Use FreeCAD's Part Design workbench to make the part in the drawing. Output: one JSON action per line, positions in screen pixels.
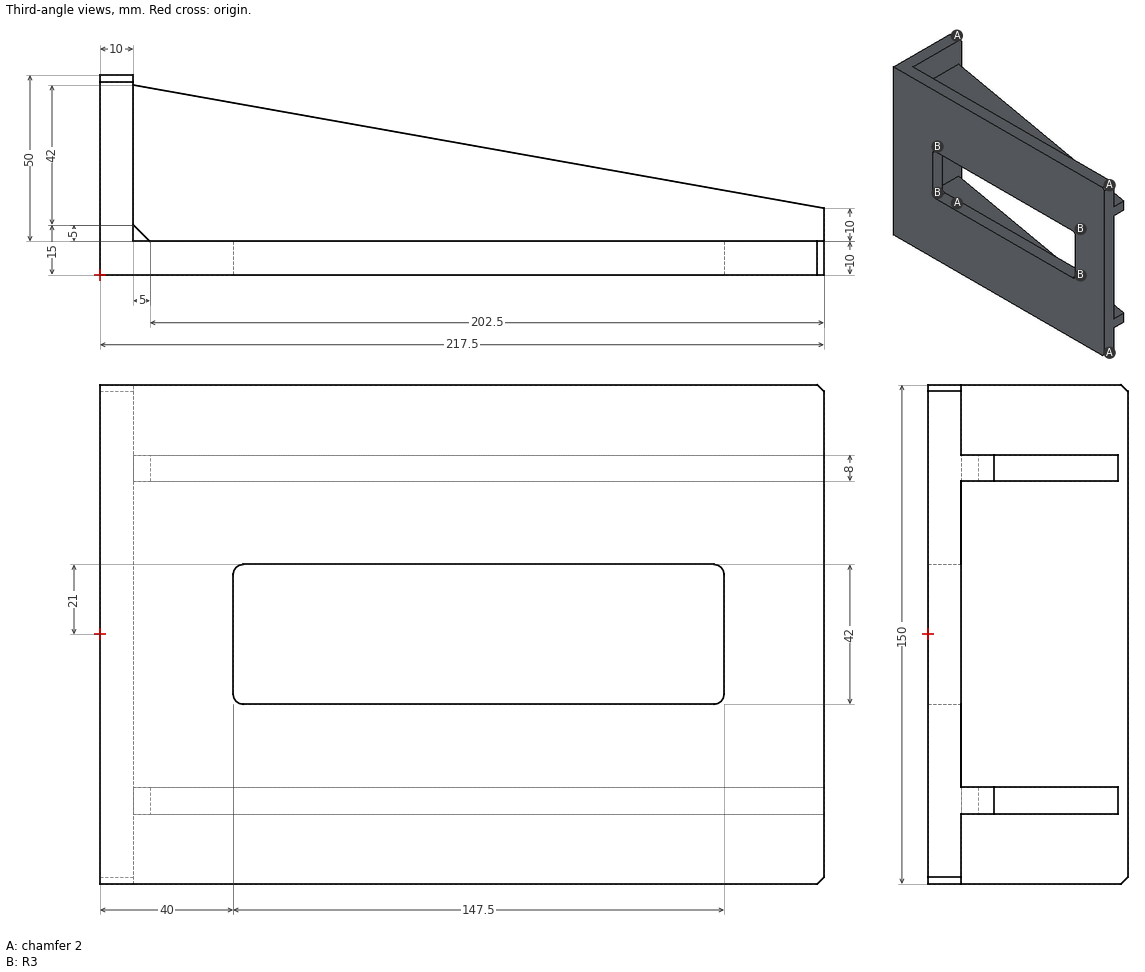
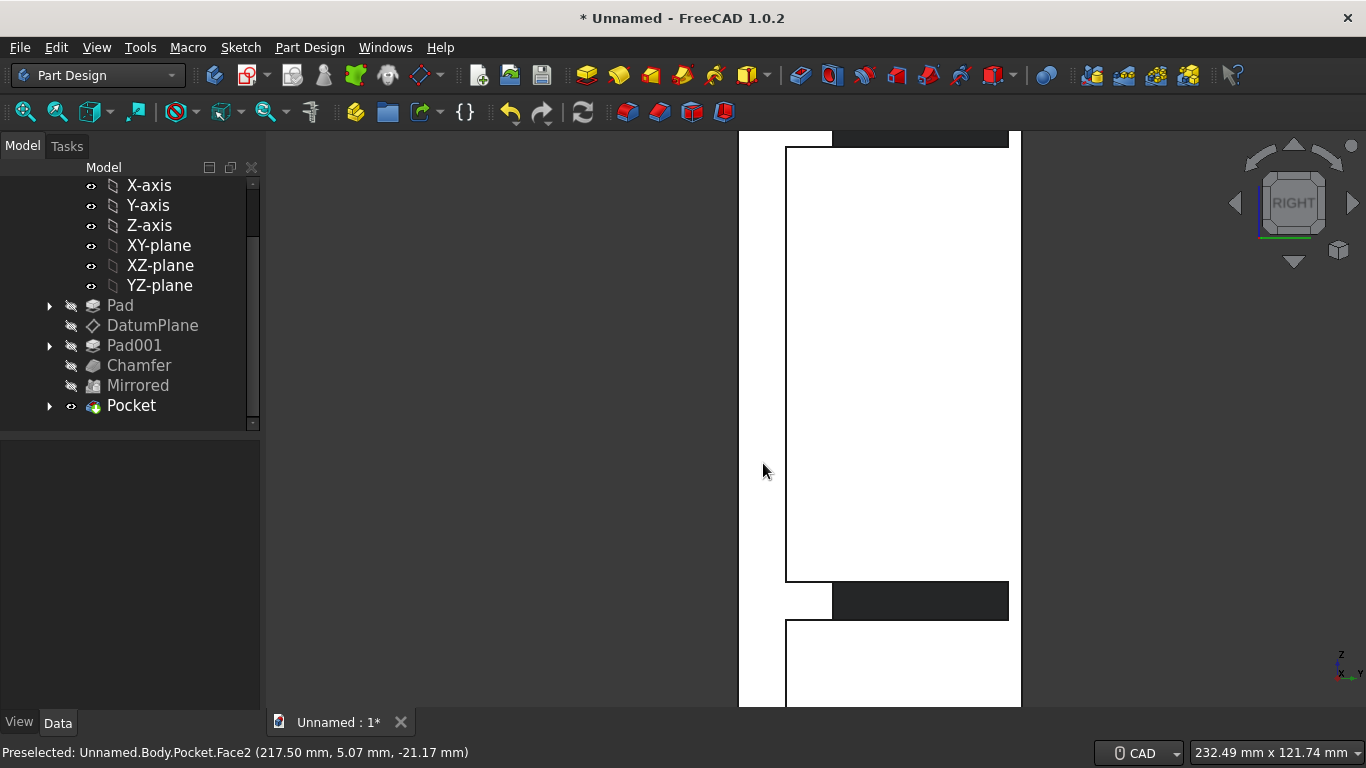
{"action": "left_click", "coordinate": [26, 112]}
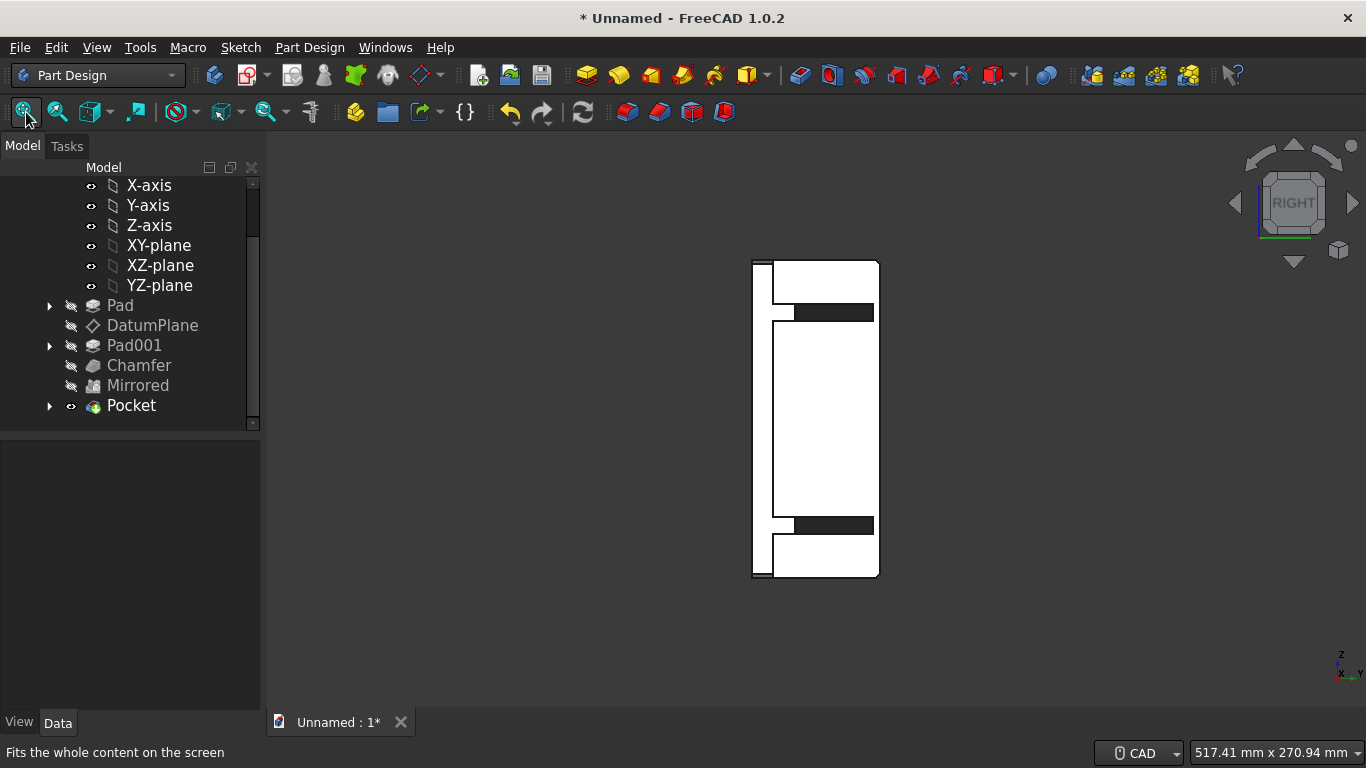
{"action": "key", "text": "5"}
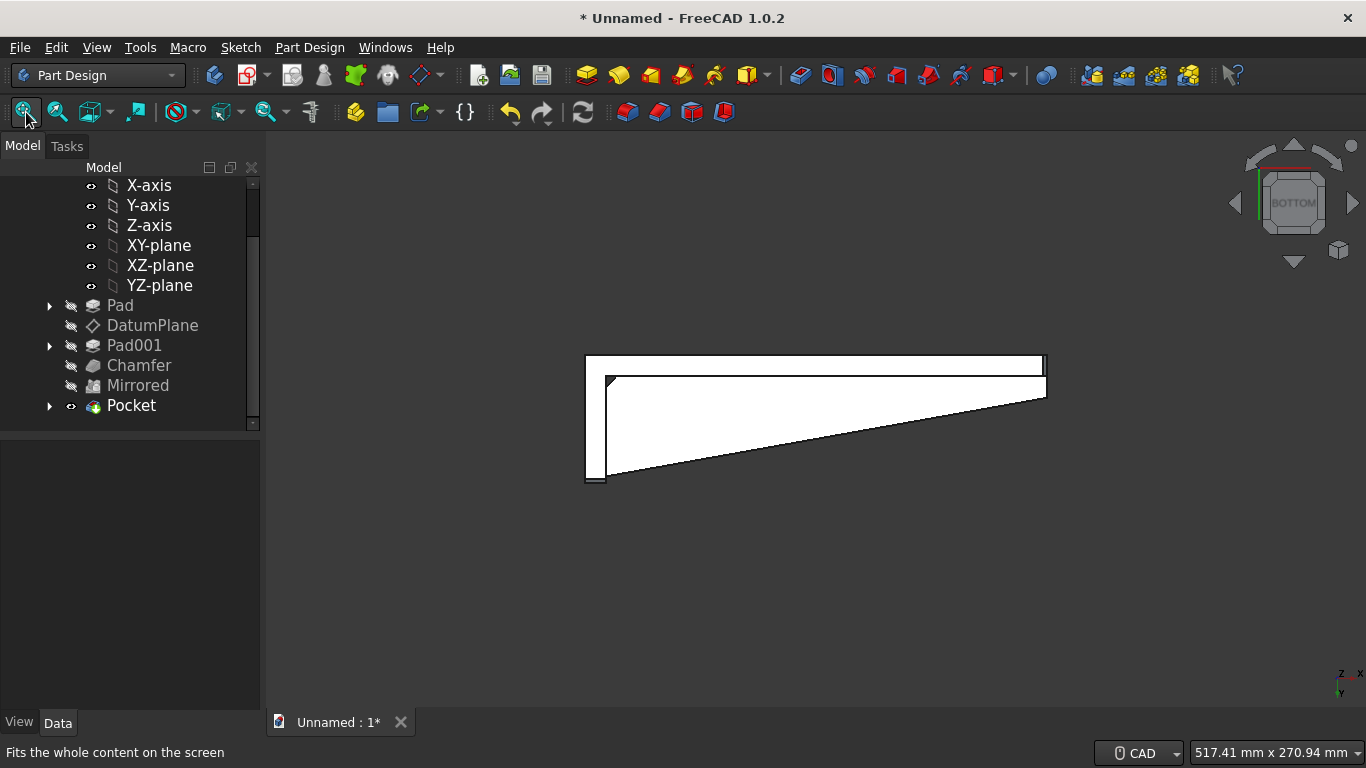
{"action": "left_click", "coordinate": [26, 112]}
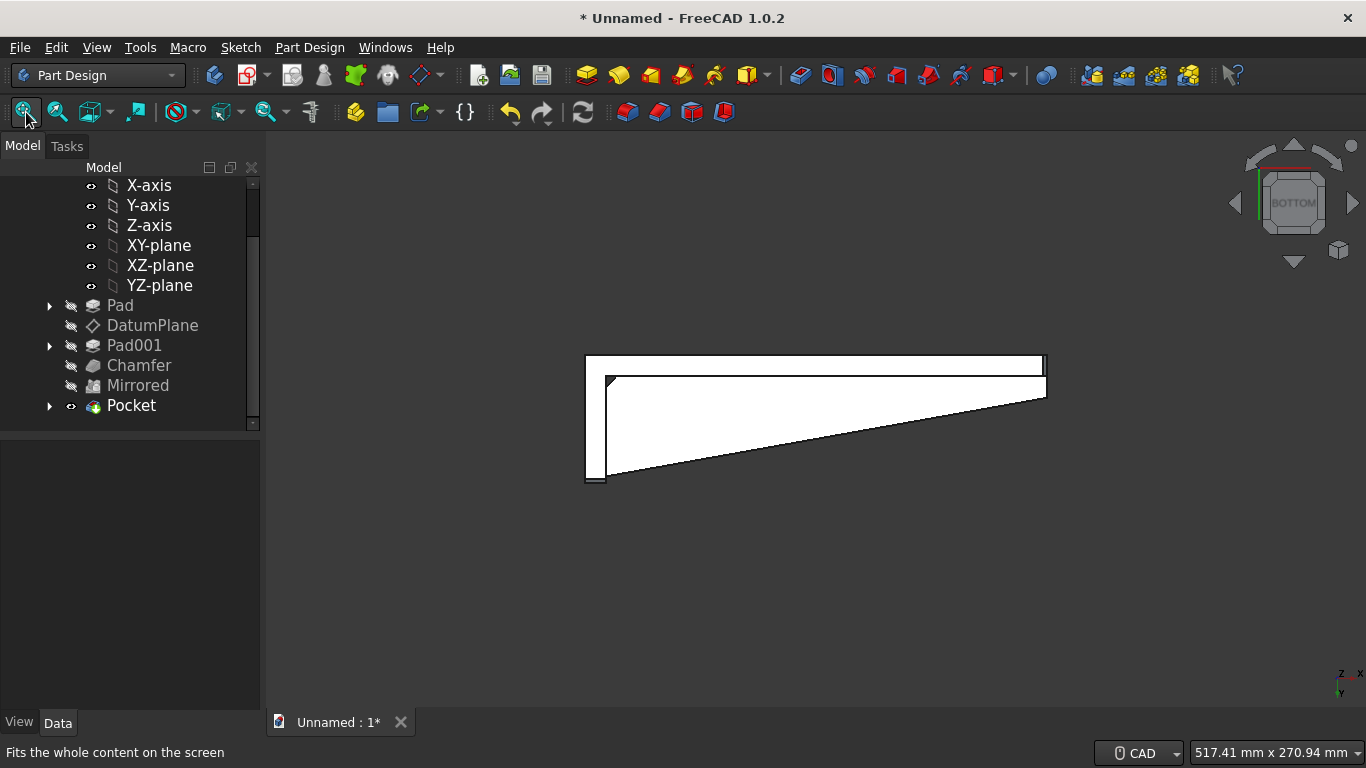
{"action": "scroll", "coordinate": [983, 365], "scroll_direction": "up", "scroll_amount": 4}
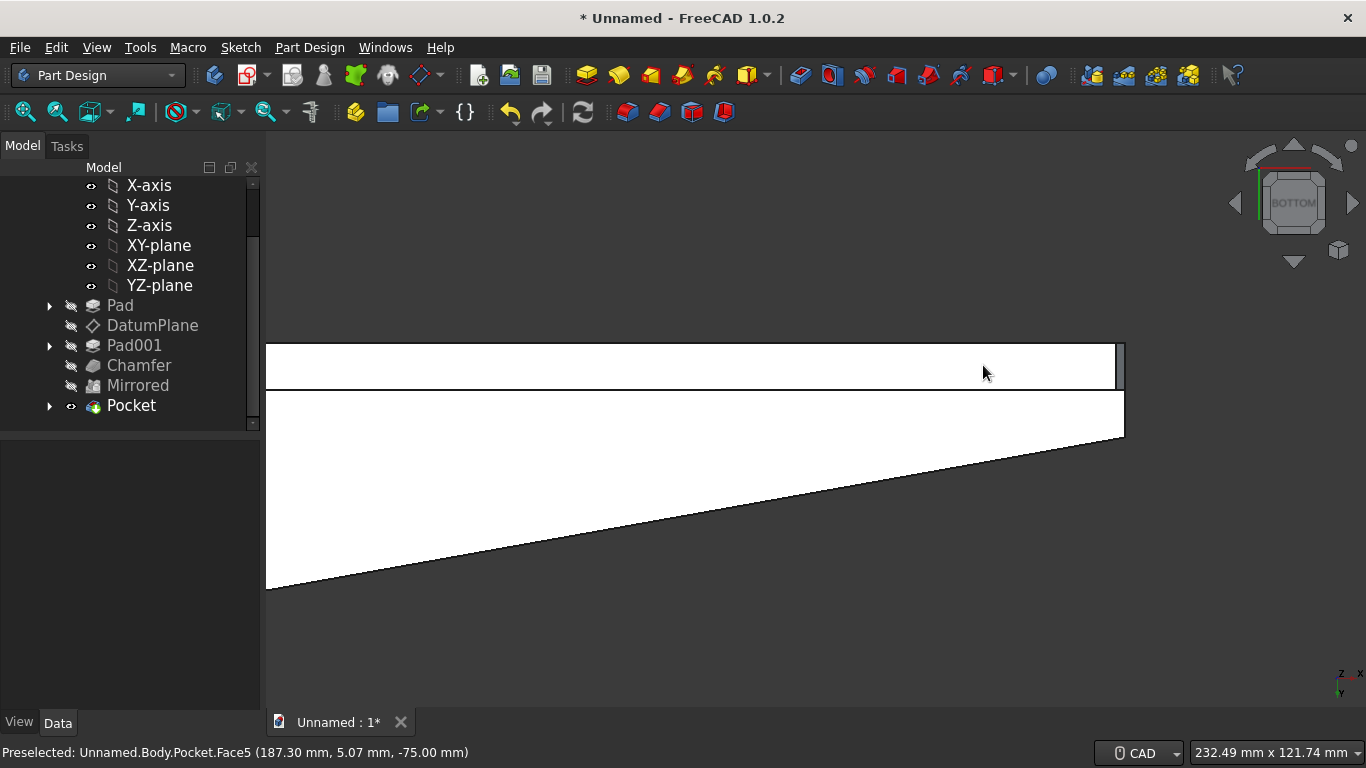
{"action": "left_click", "coordinate": [26, 112]}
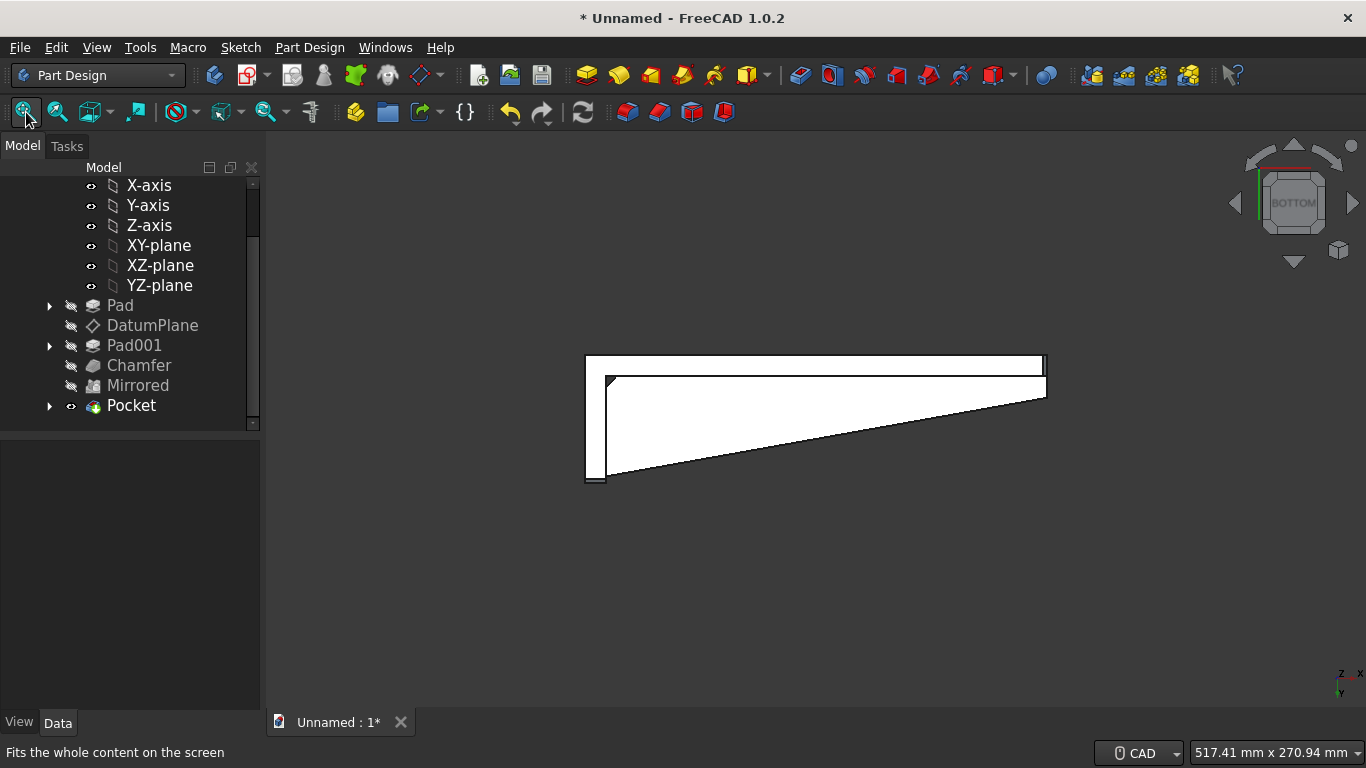
{"action": "key", "text": "4"}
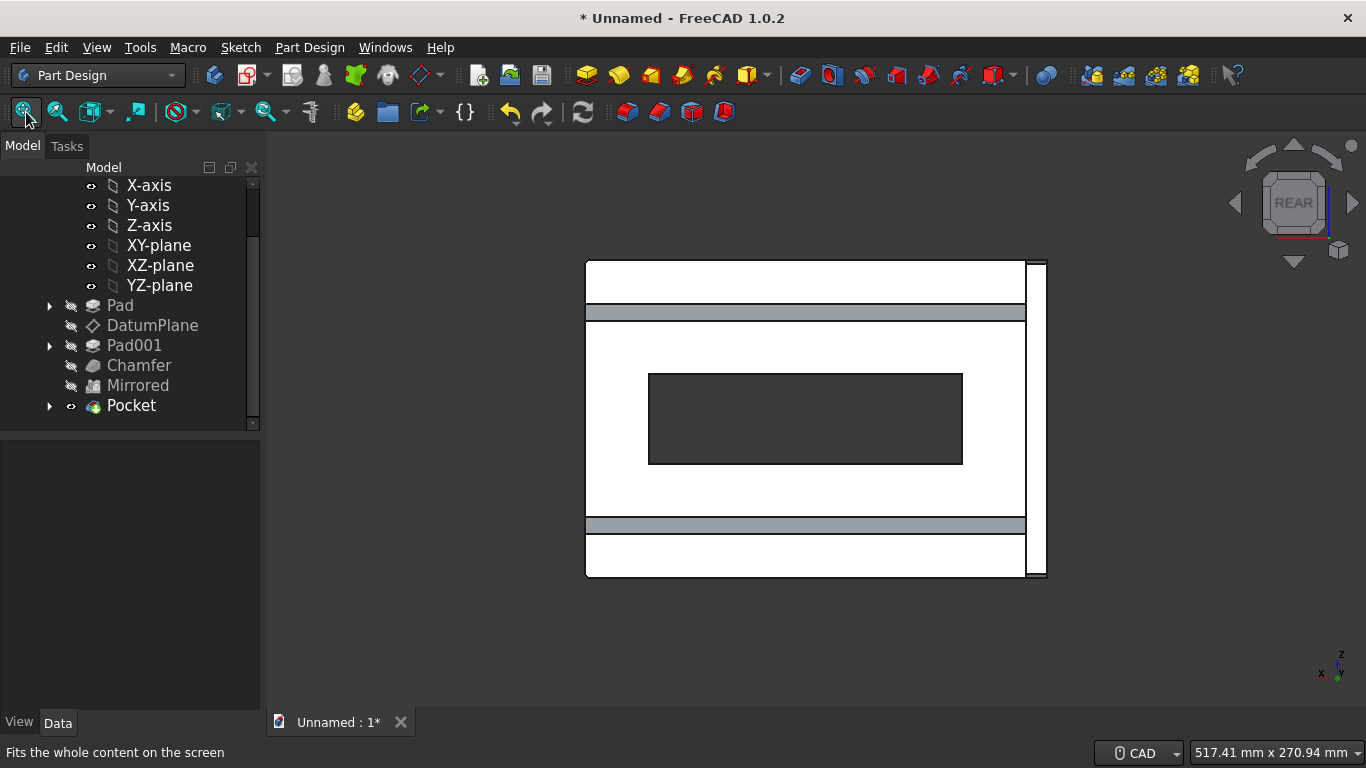
{"action": "scroll", "coordinate": [649, 463], "scroll_direction": "up", "scroll_amount": 4}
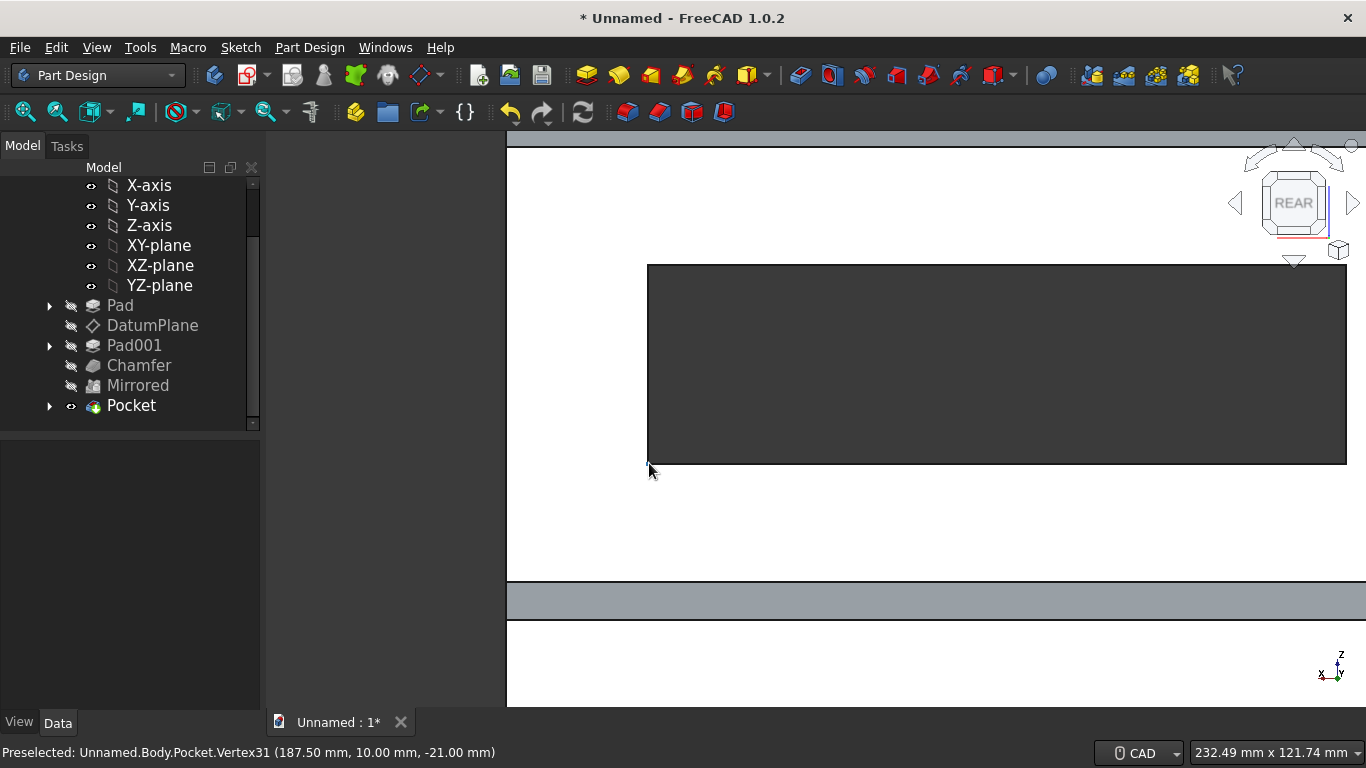
{"action": "left_click", "coordinate": [26, 112]}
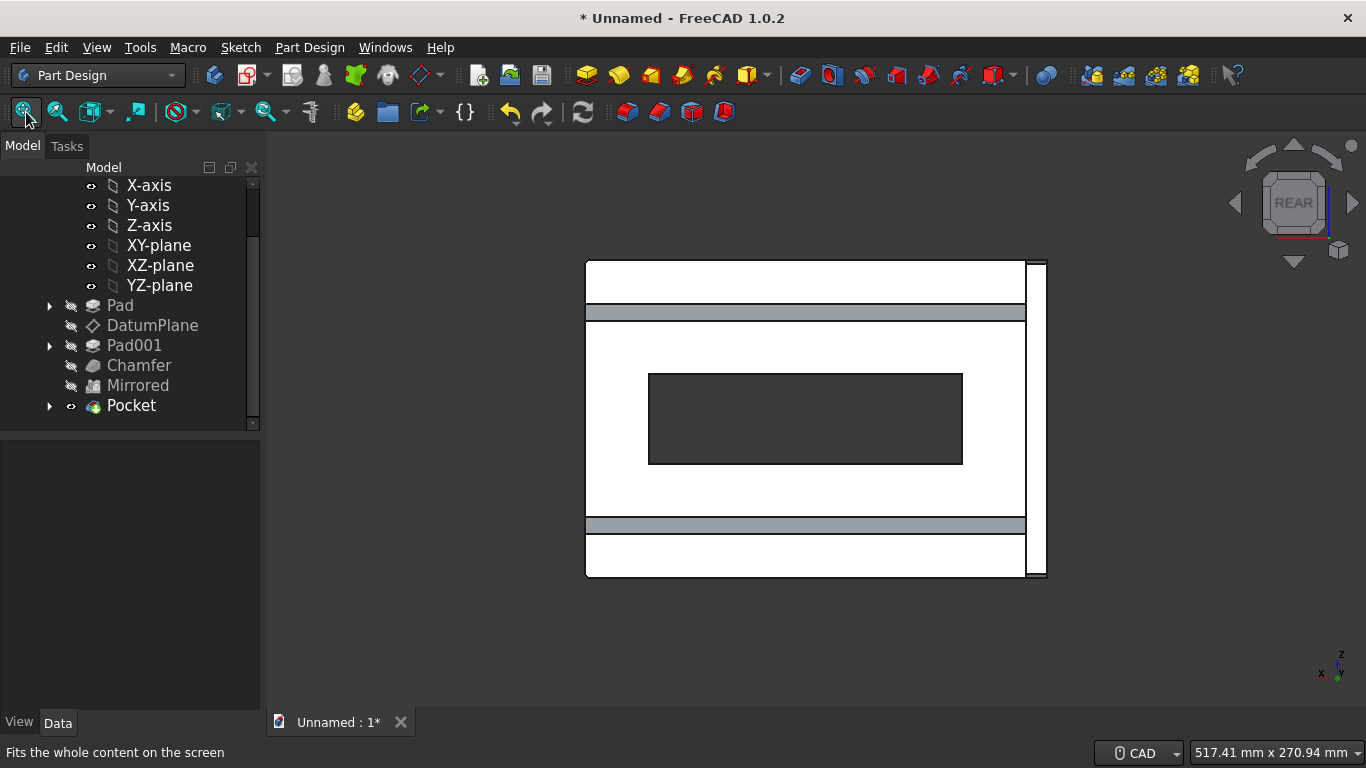
{"action": "key", "text": "6"}